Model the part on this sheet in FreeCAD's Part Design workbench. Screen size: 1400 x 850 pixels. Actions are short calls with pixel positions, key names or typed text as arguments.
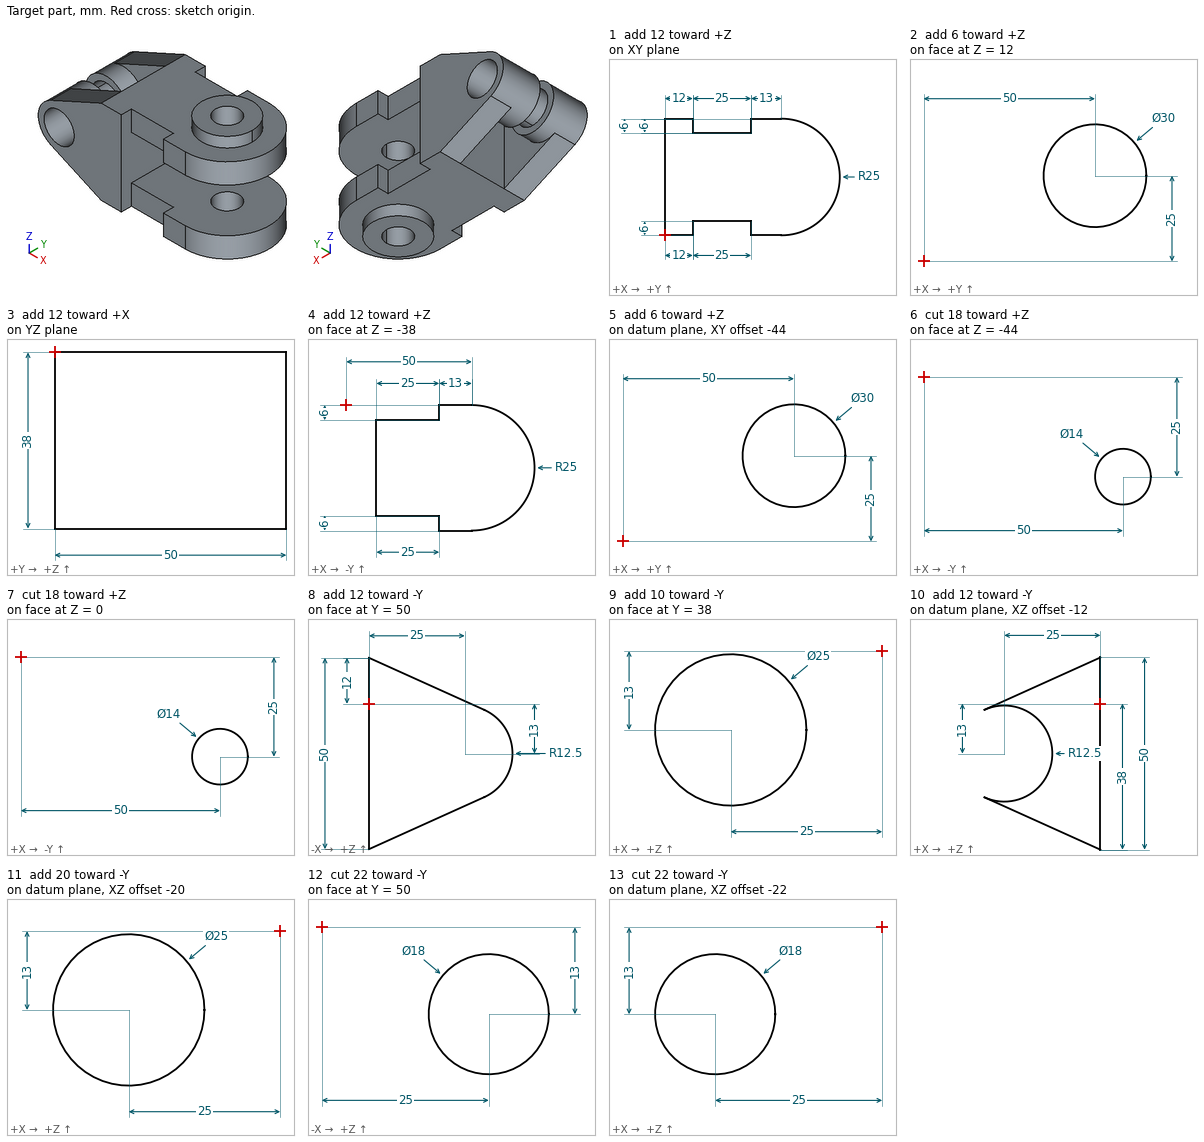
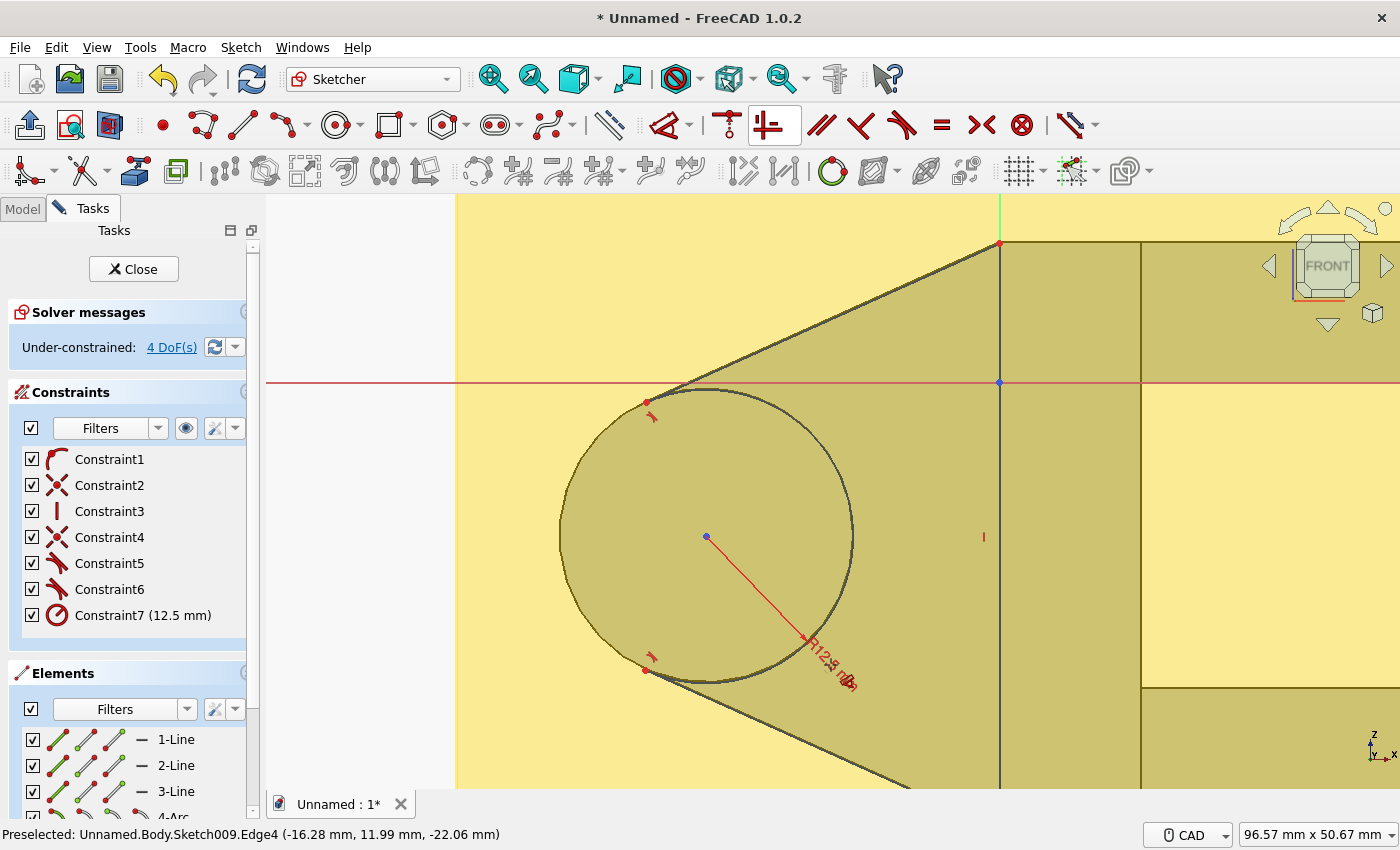
click(1000, 654)
click(1034, 502)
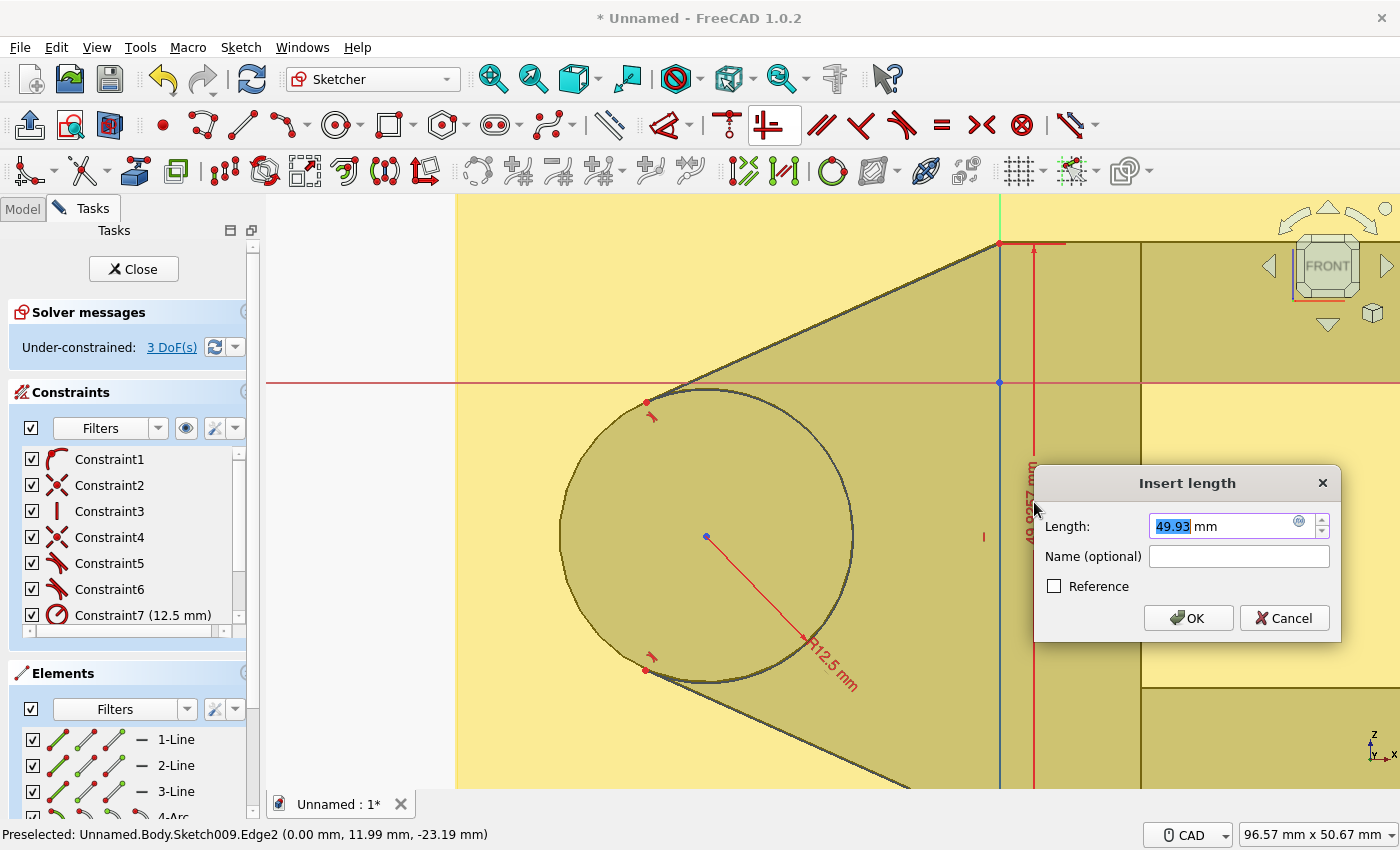
text(50)
key(Return)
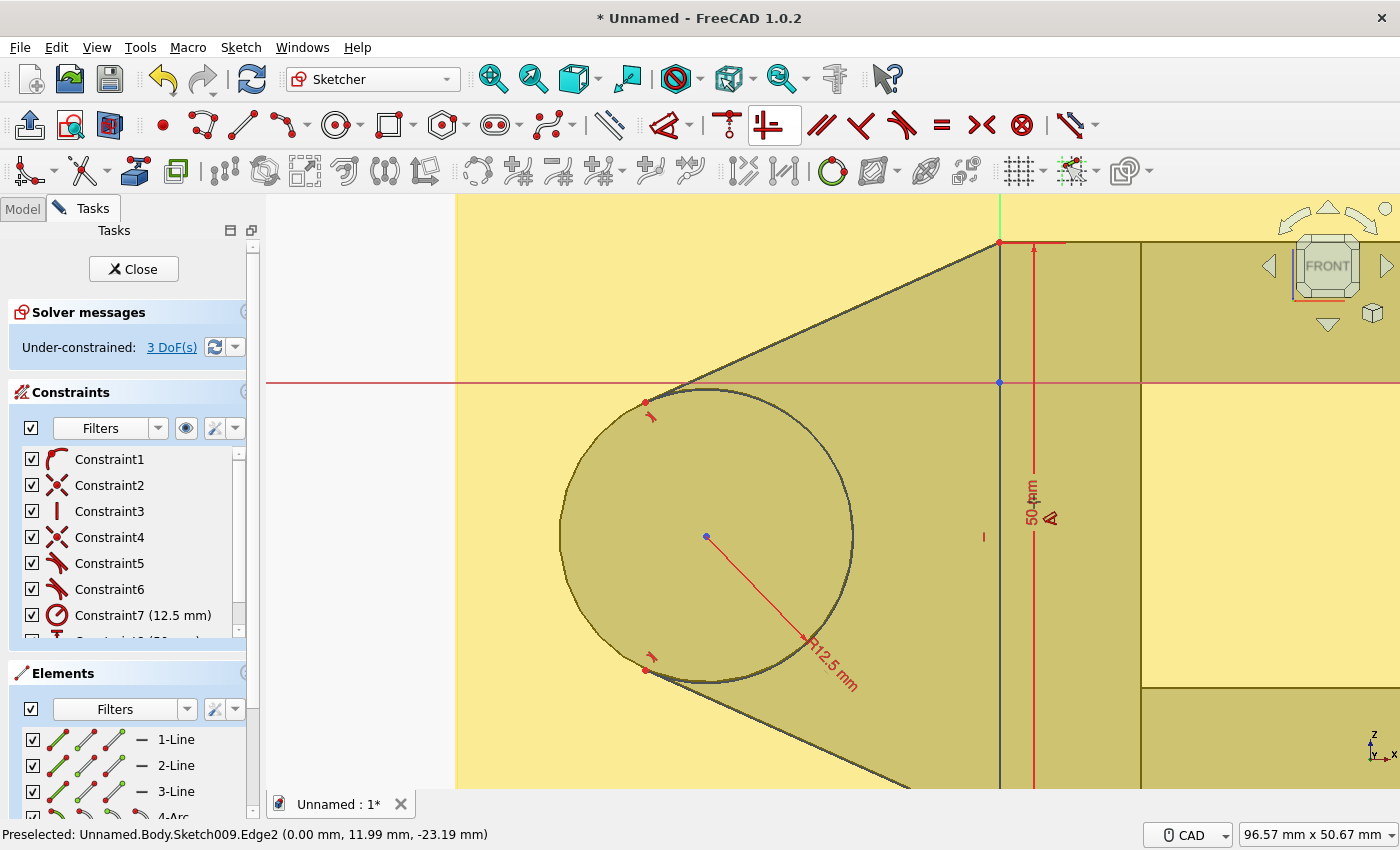
scroll(646, 402, down, 2)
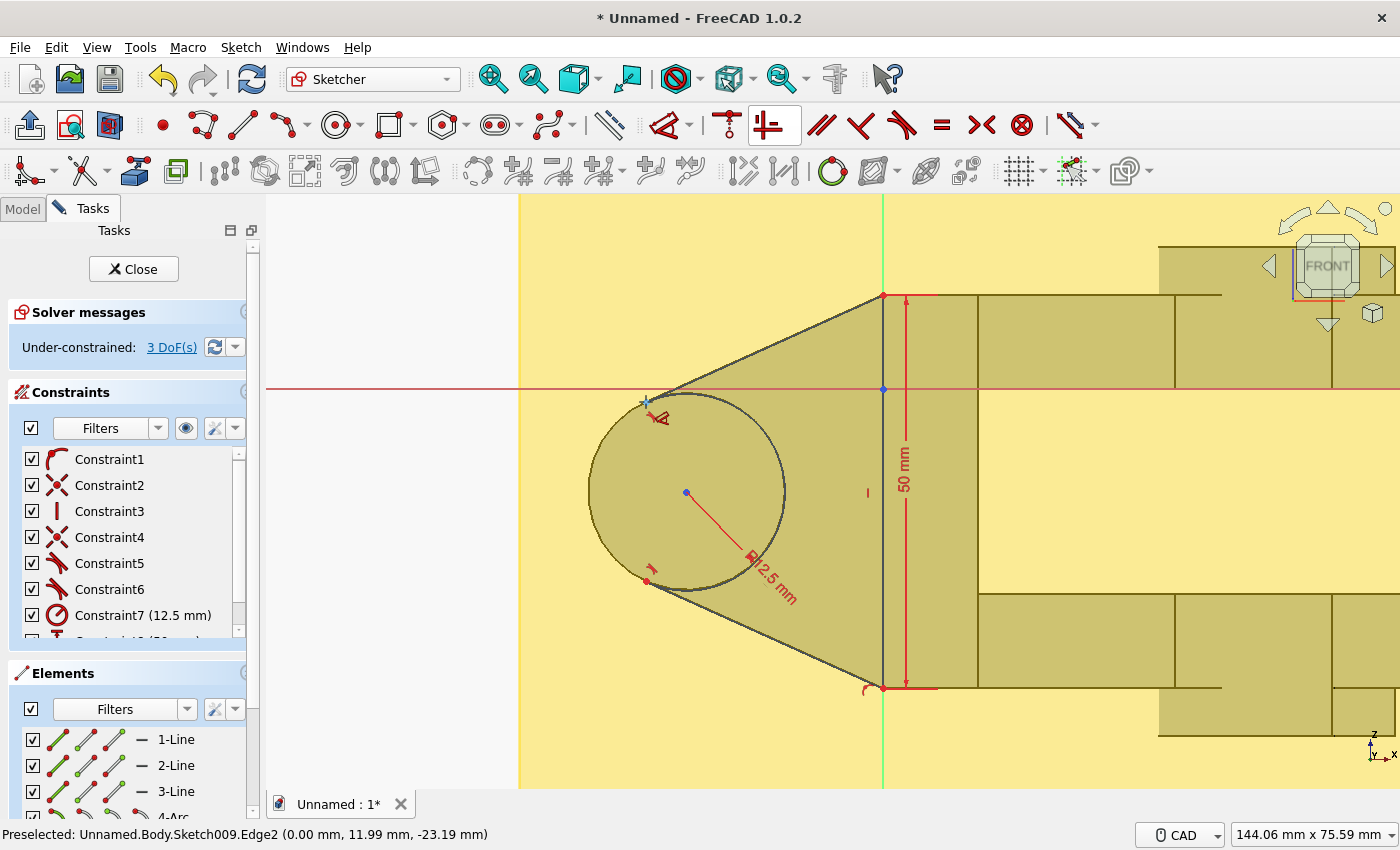
click(883, 689)
click(917, 539)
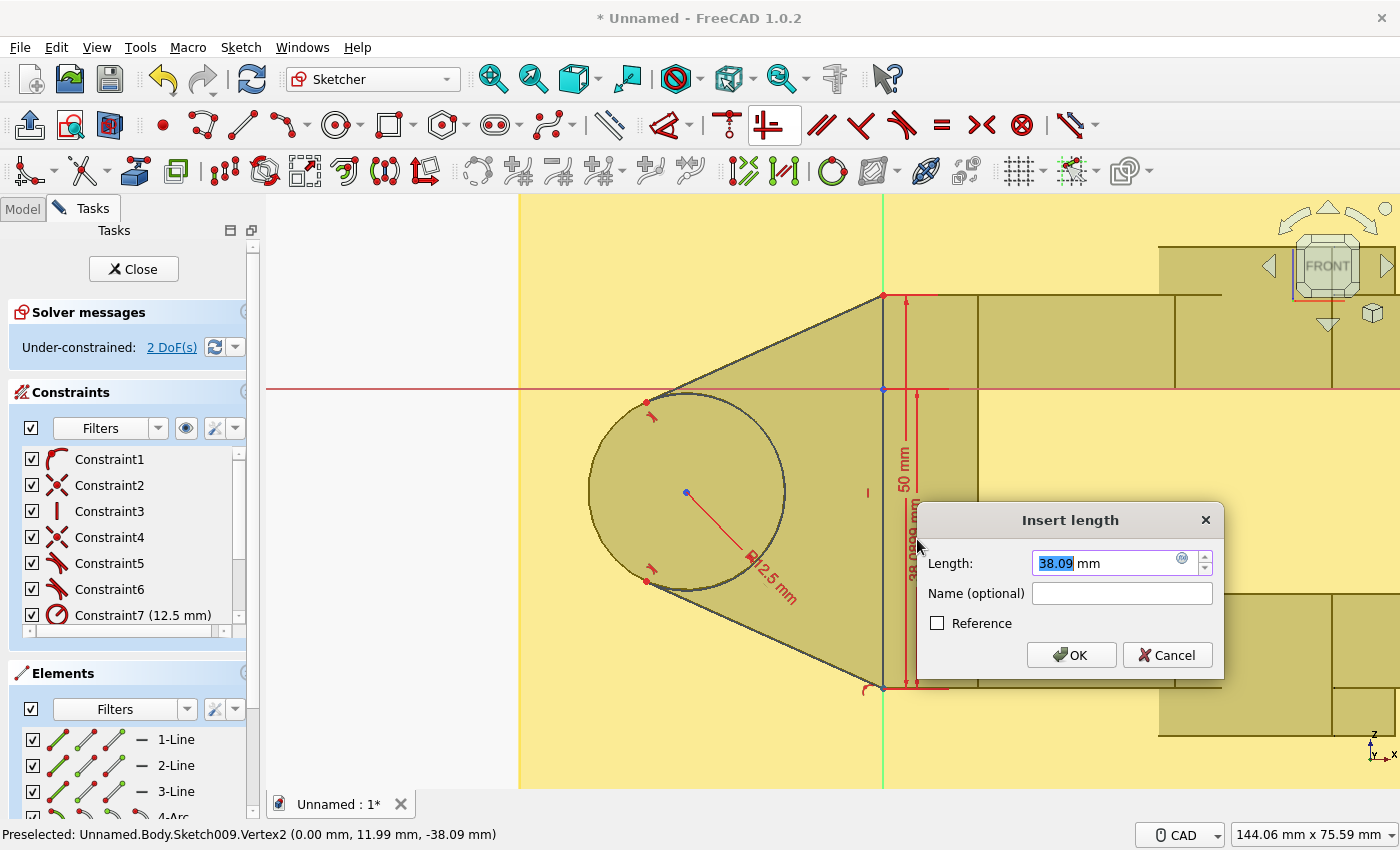
text(38)
key(Return)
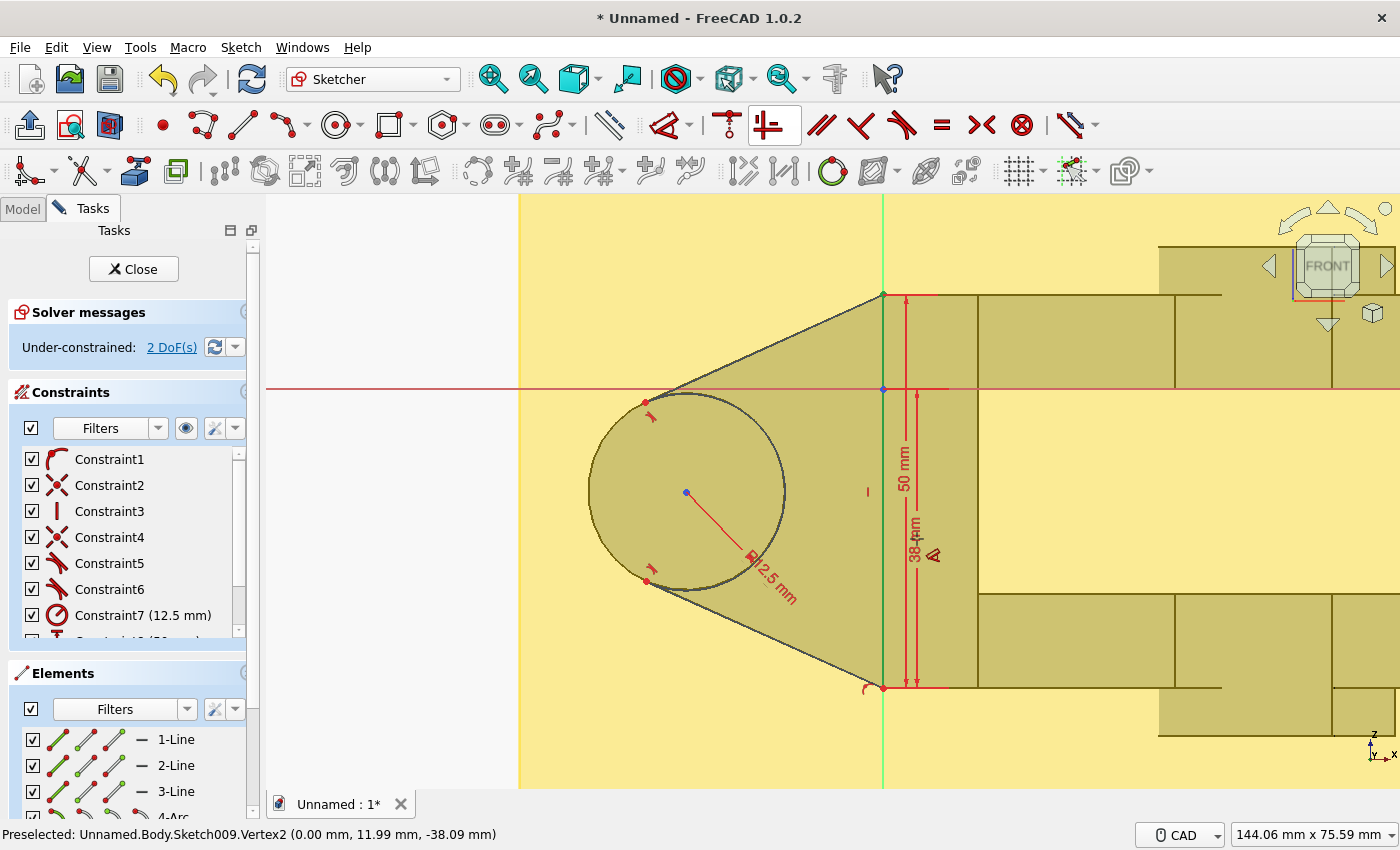
click(687, 492)
click(785, 355)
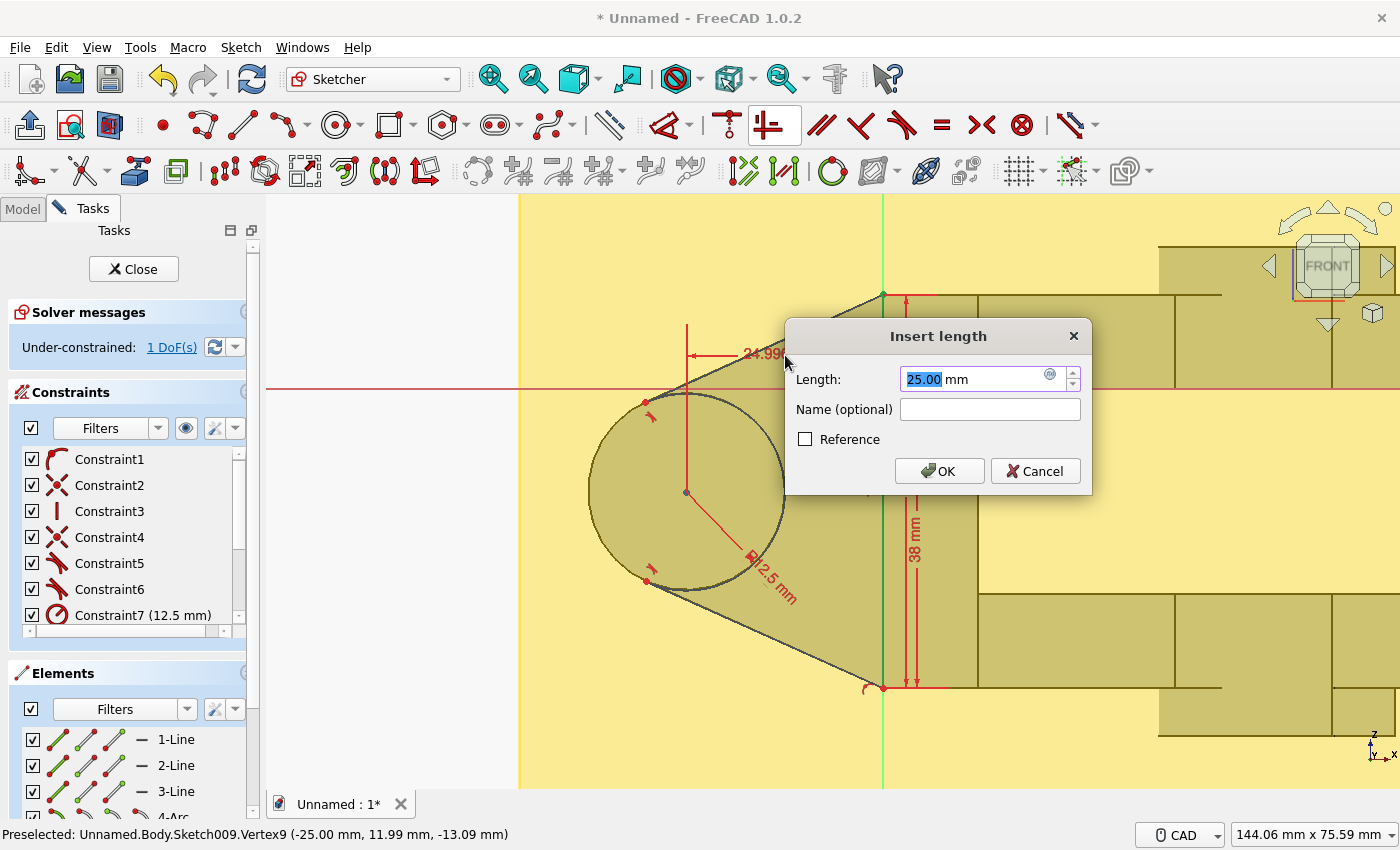
text(25)
key(Return)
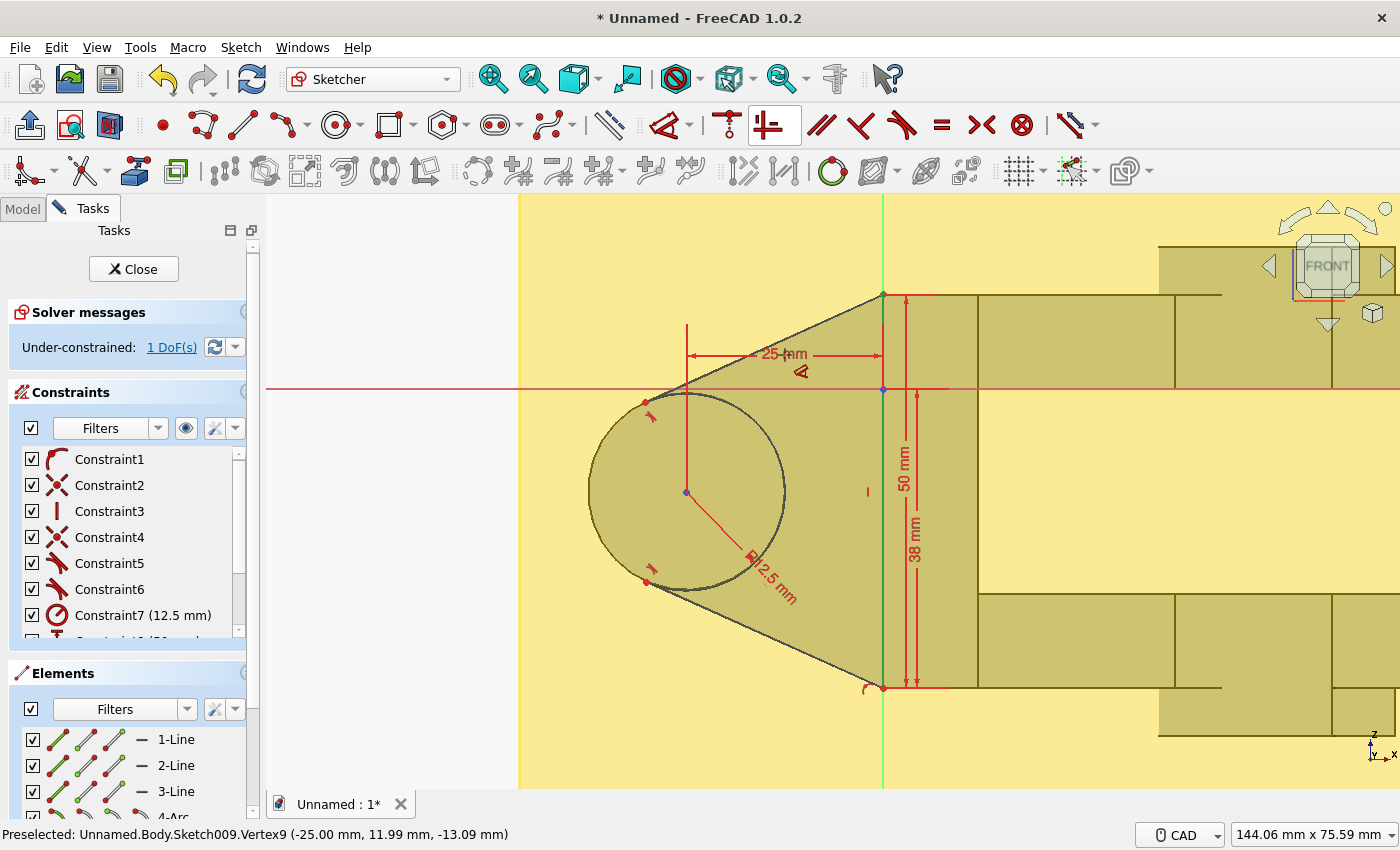
click(687, 492)
click(917, 441)